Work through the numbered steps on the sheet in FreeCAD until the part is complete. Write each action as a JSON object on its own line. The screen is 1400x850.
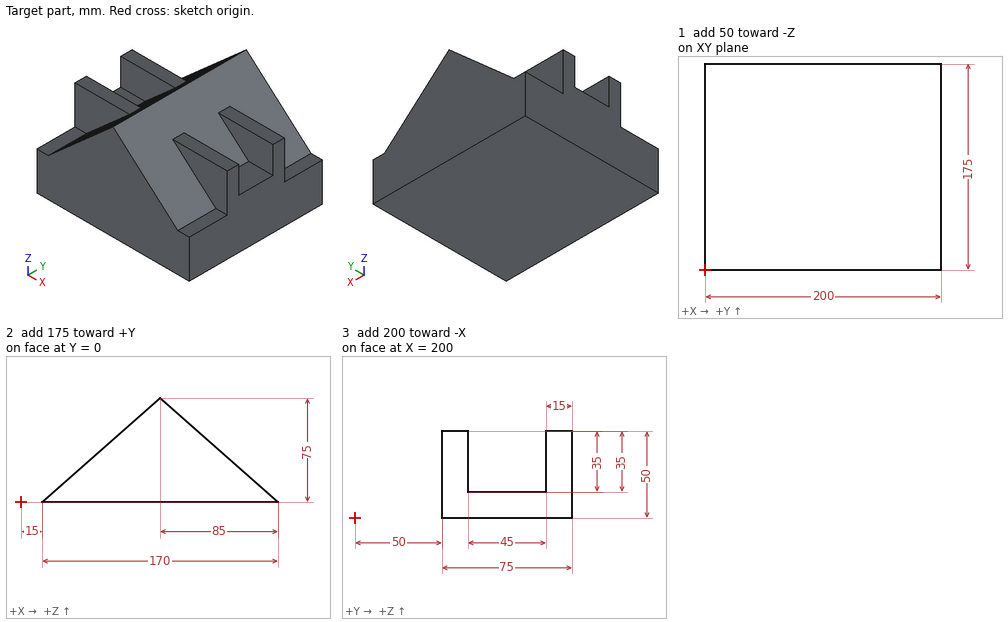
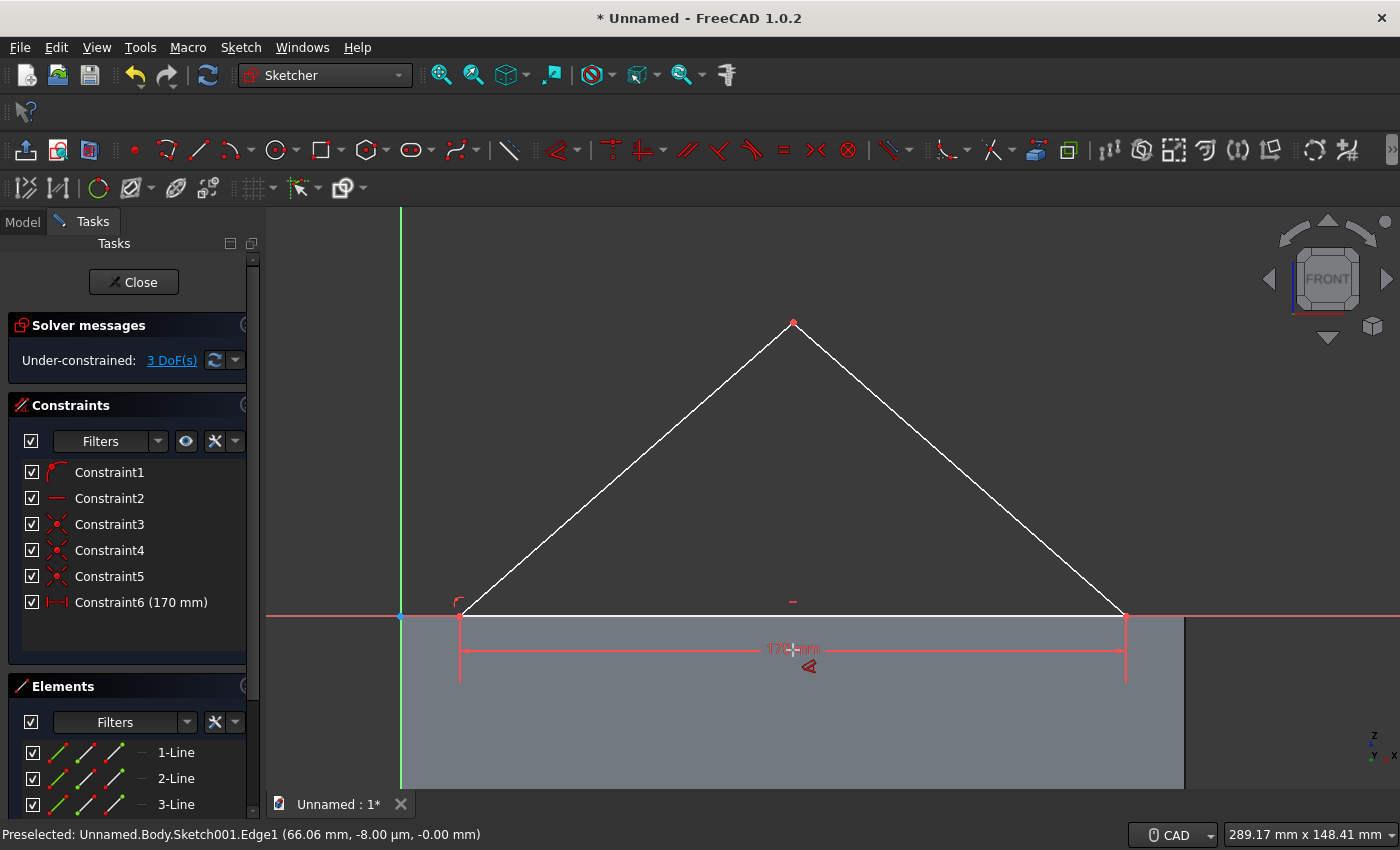
{"action": "left_click", "coordinate": [460, 616]}
{"action": "left_click", "coordinate": [430, 650]}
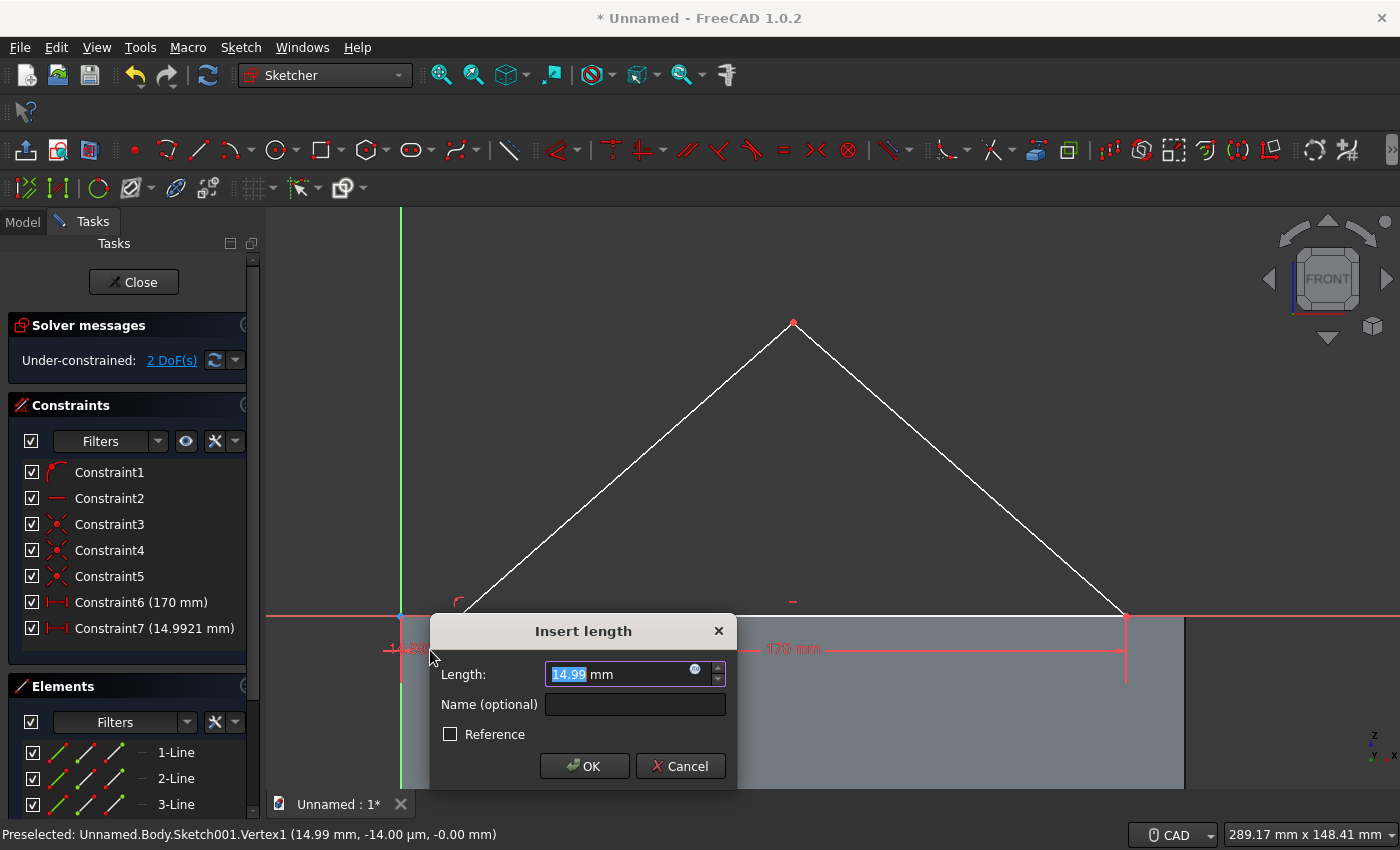
{"action": "type", "text": "15"}
{"action": "key", "text": "Return"}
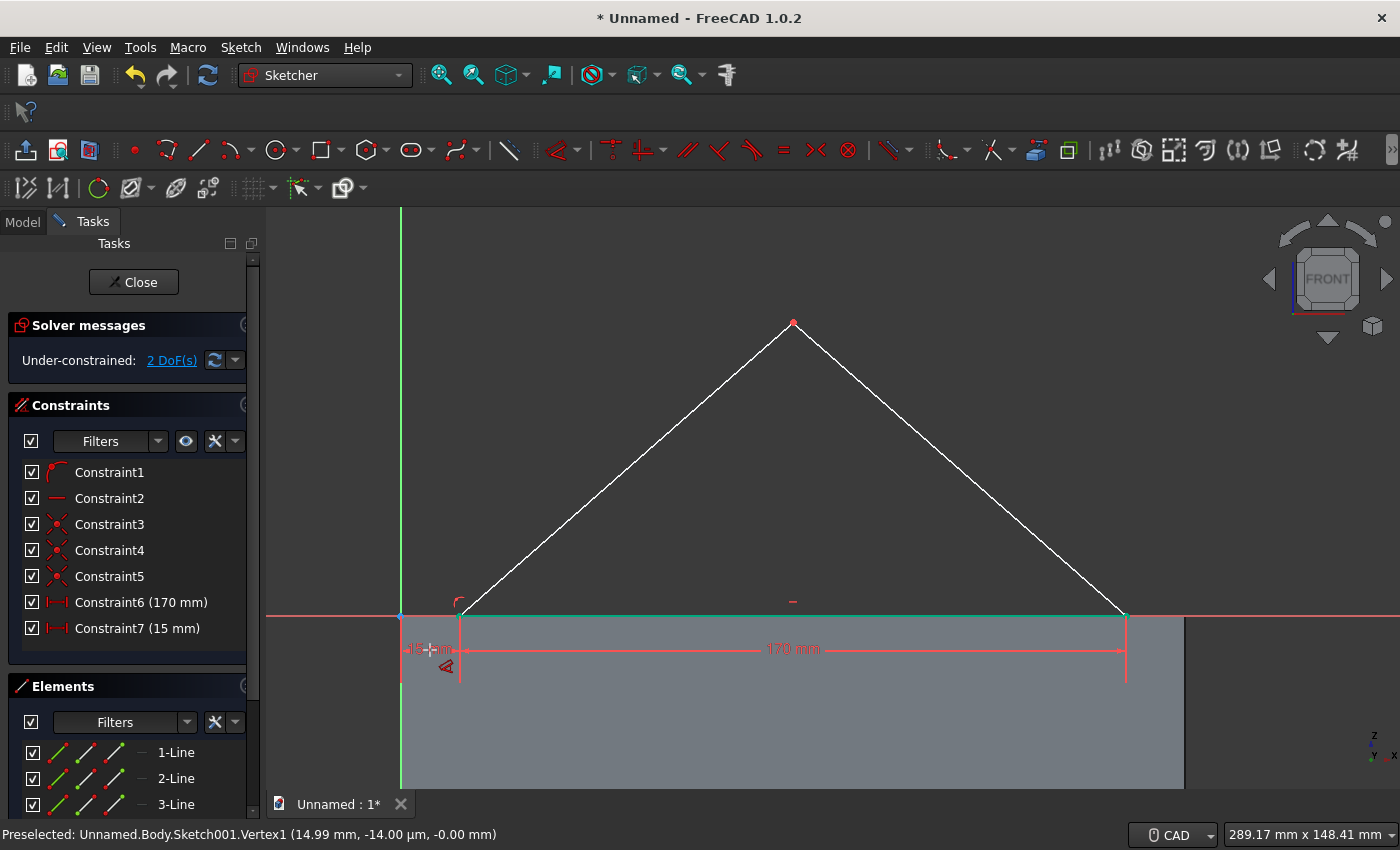
{"action": "left_click", "coordinate": [793, 323]}
{"action": "left_click", "coordinate": [367, 470]}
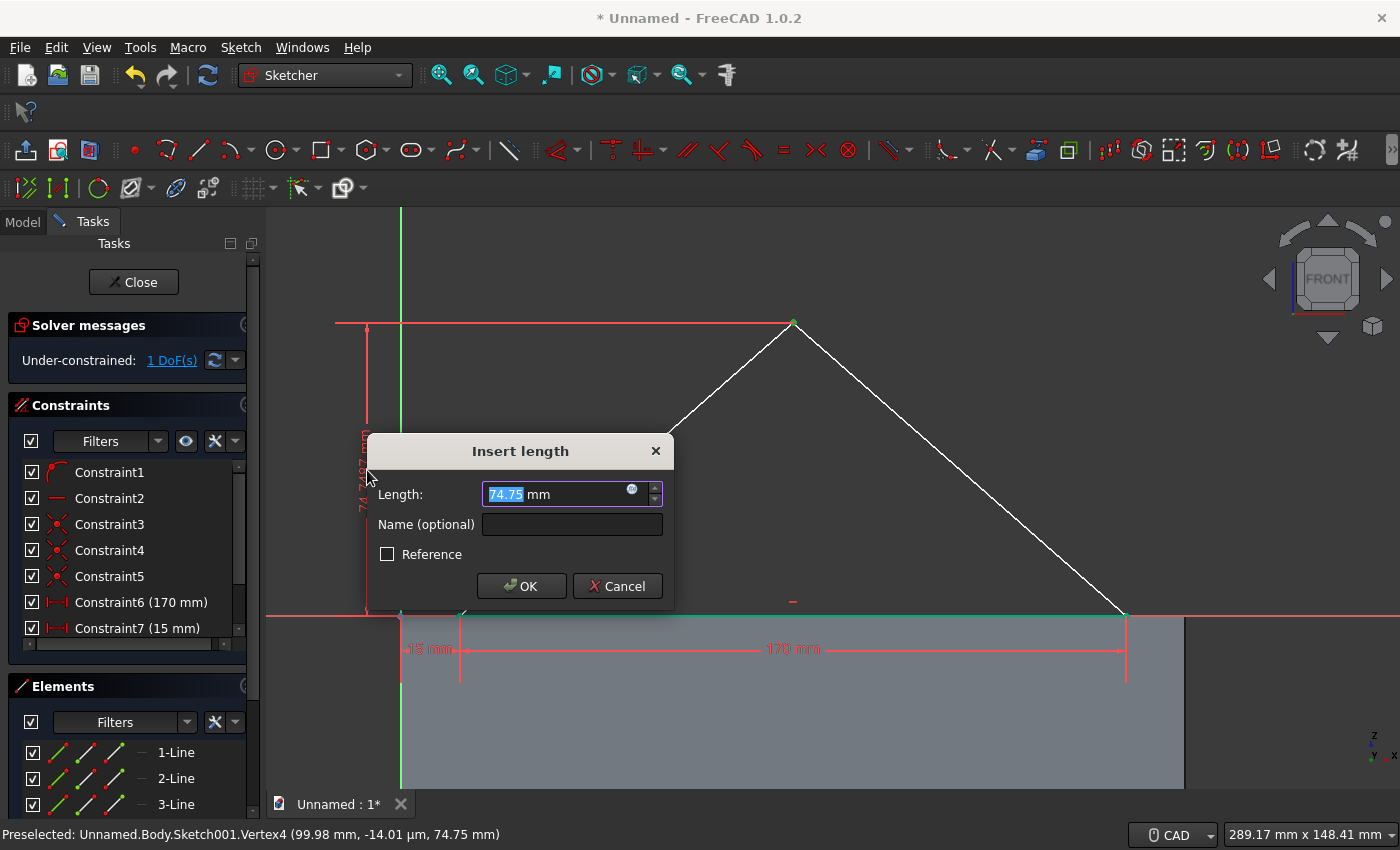
{"action": "type", "text": "75"}
{"action": "key", "text": "Return"}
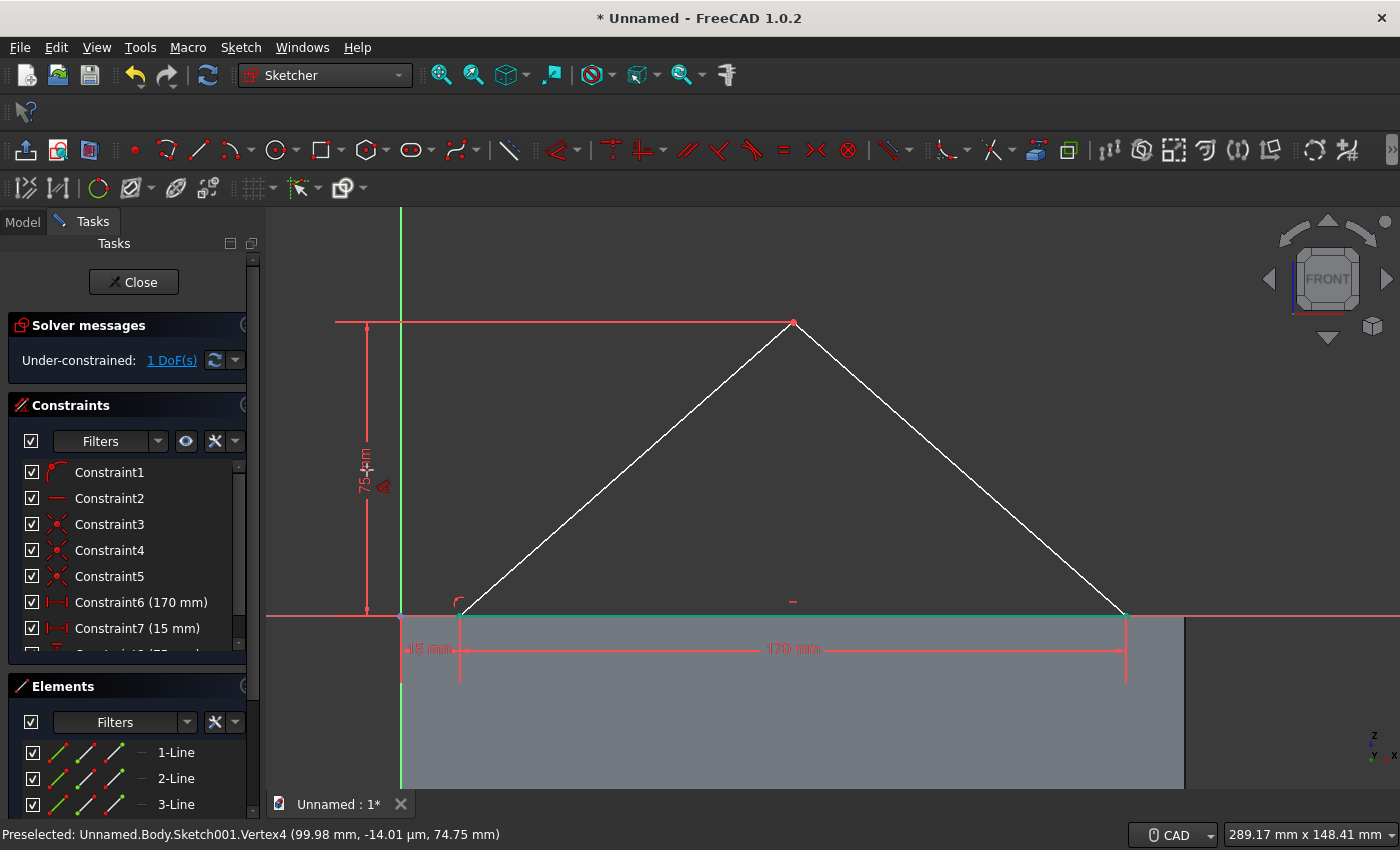
{"action": "left_click", "coordinate": [1026, 528]}
{"action": "left_click", "coordinate": [960, 650]}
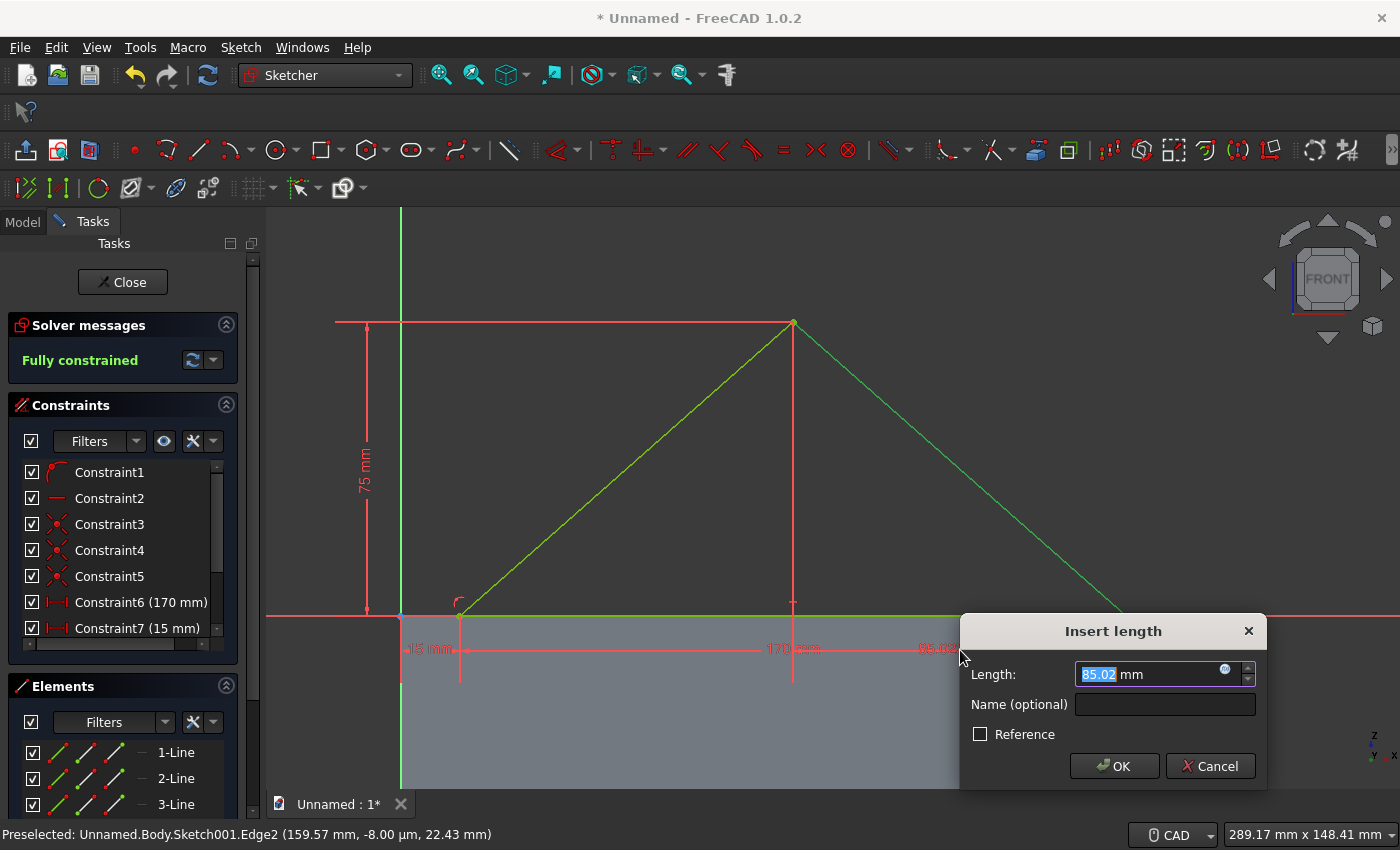
{"action": "type", "text": "85"}
{"action": "key", "text": "Return"}
{"action": "key", "text": "Escape"}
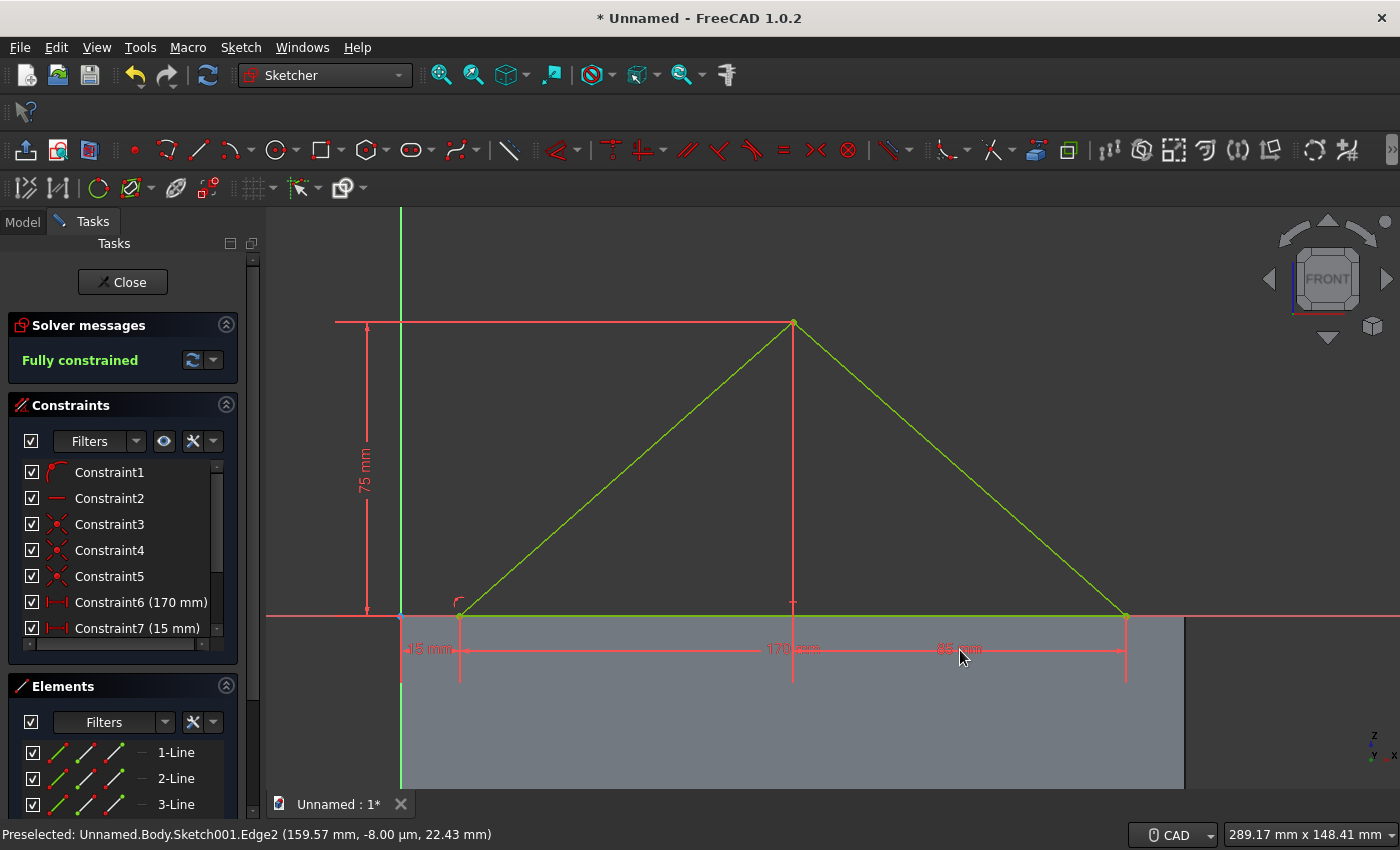
{"action": "left_click", "coordinate": [123, 282]}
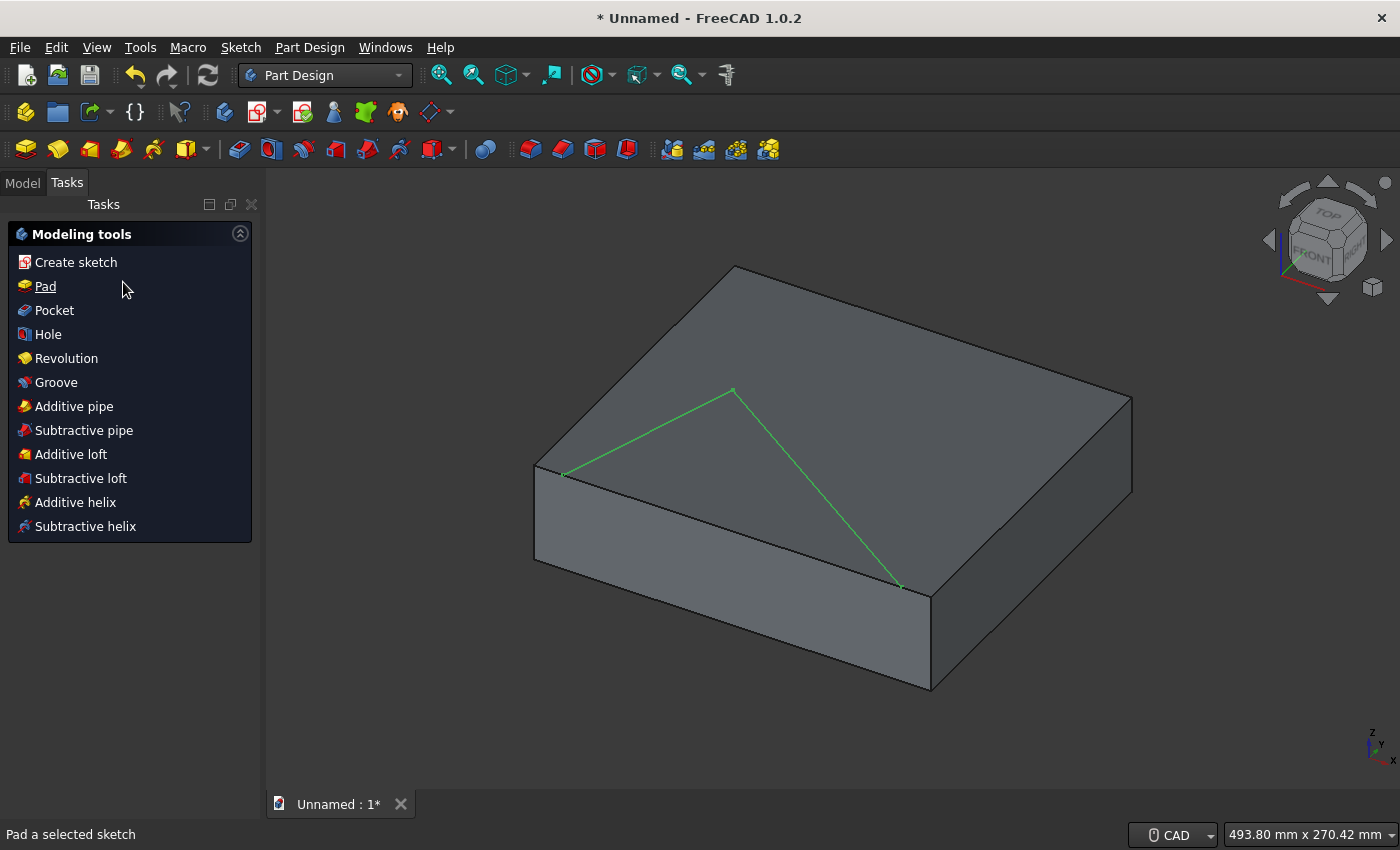
{"action": "left_click", "coordinate": [26, 150]}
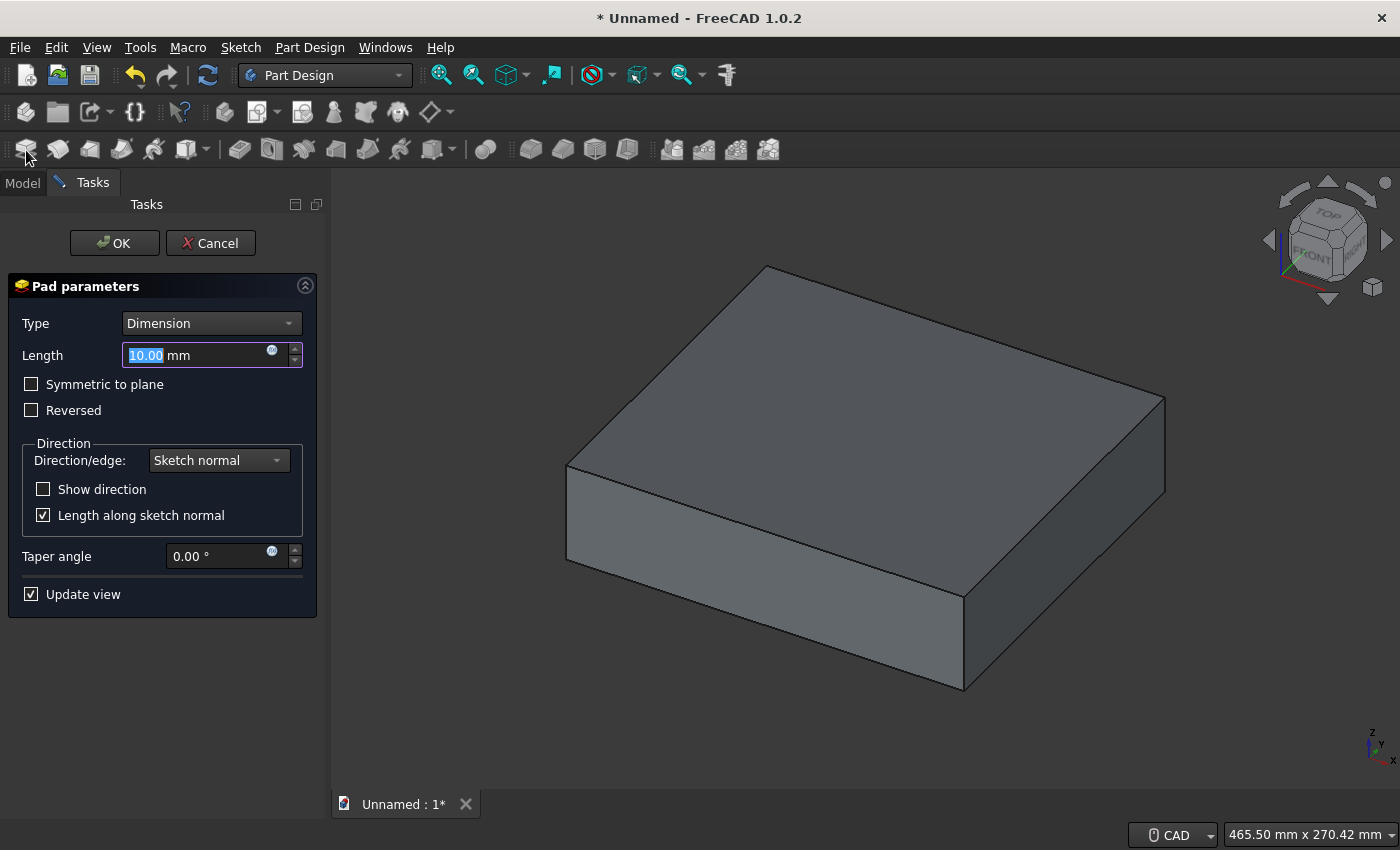
{"action": "type", "text": "175"}
{"action": "key", "text": "Tab"}